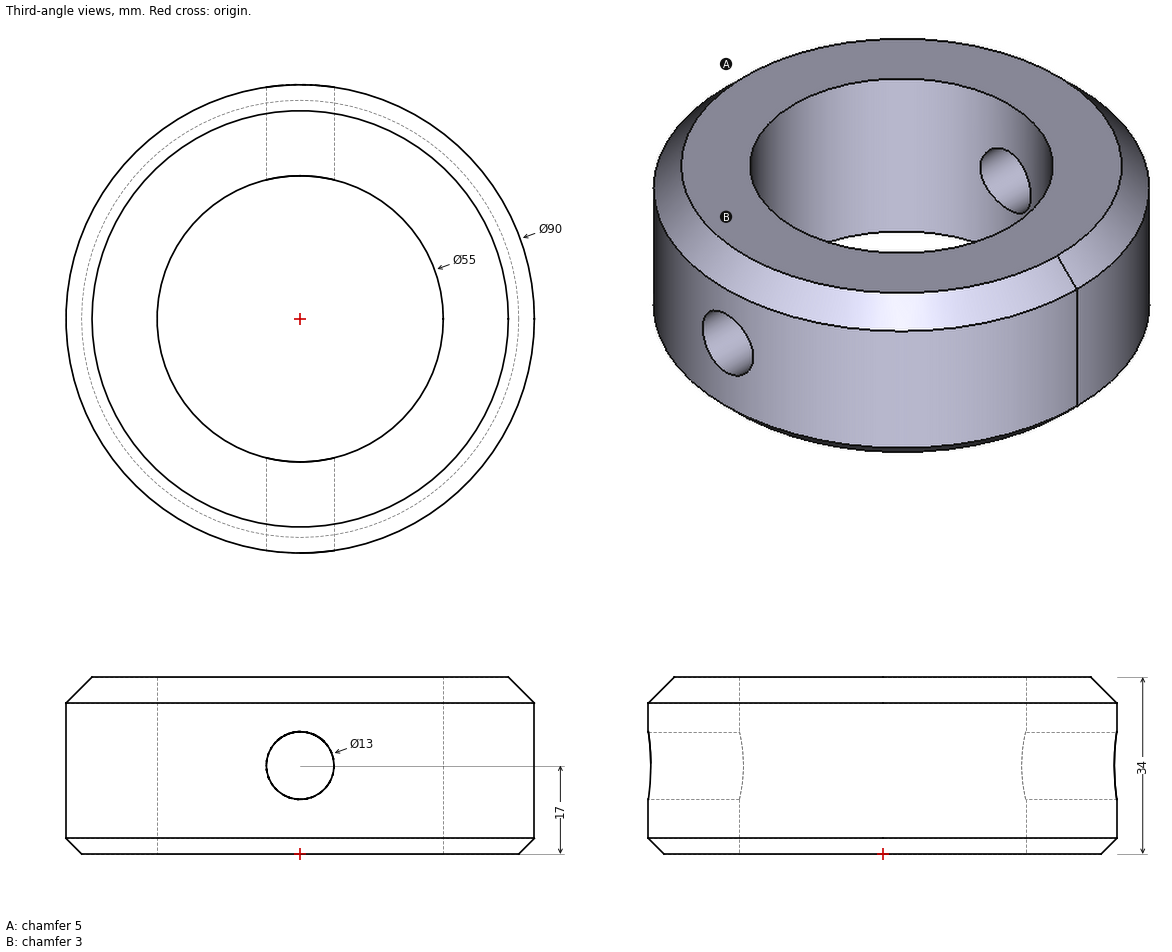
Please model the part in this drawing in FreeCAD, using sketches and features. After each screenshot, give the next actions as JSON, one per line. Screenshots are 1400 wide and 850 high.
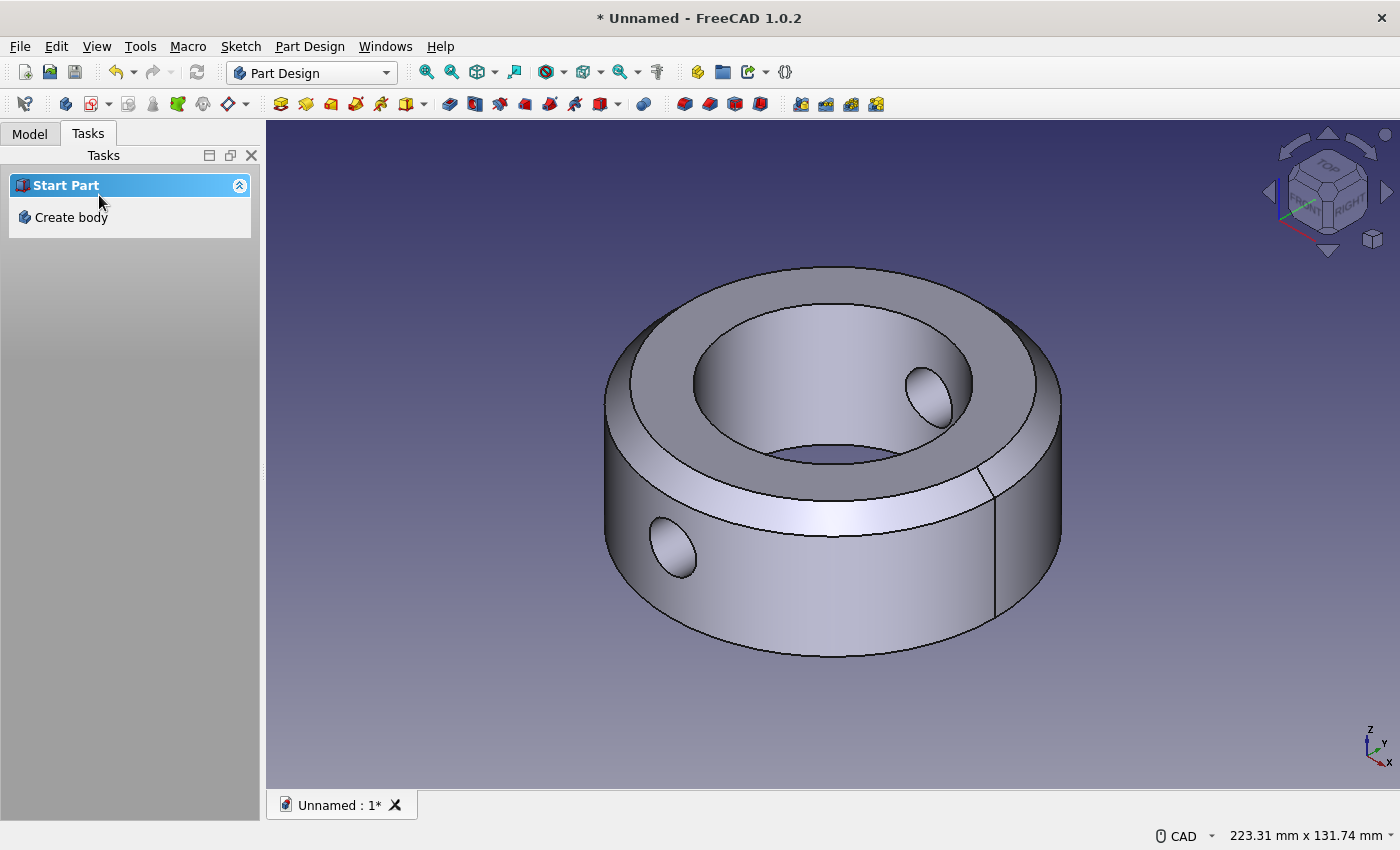
{"action": "left_click", "coordinate": [729, 642]}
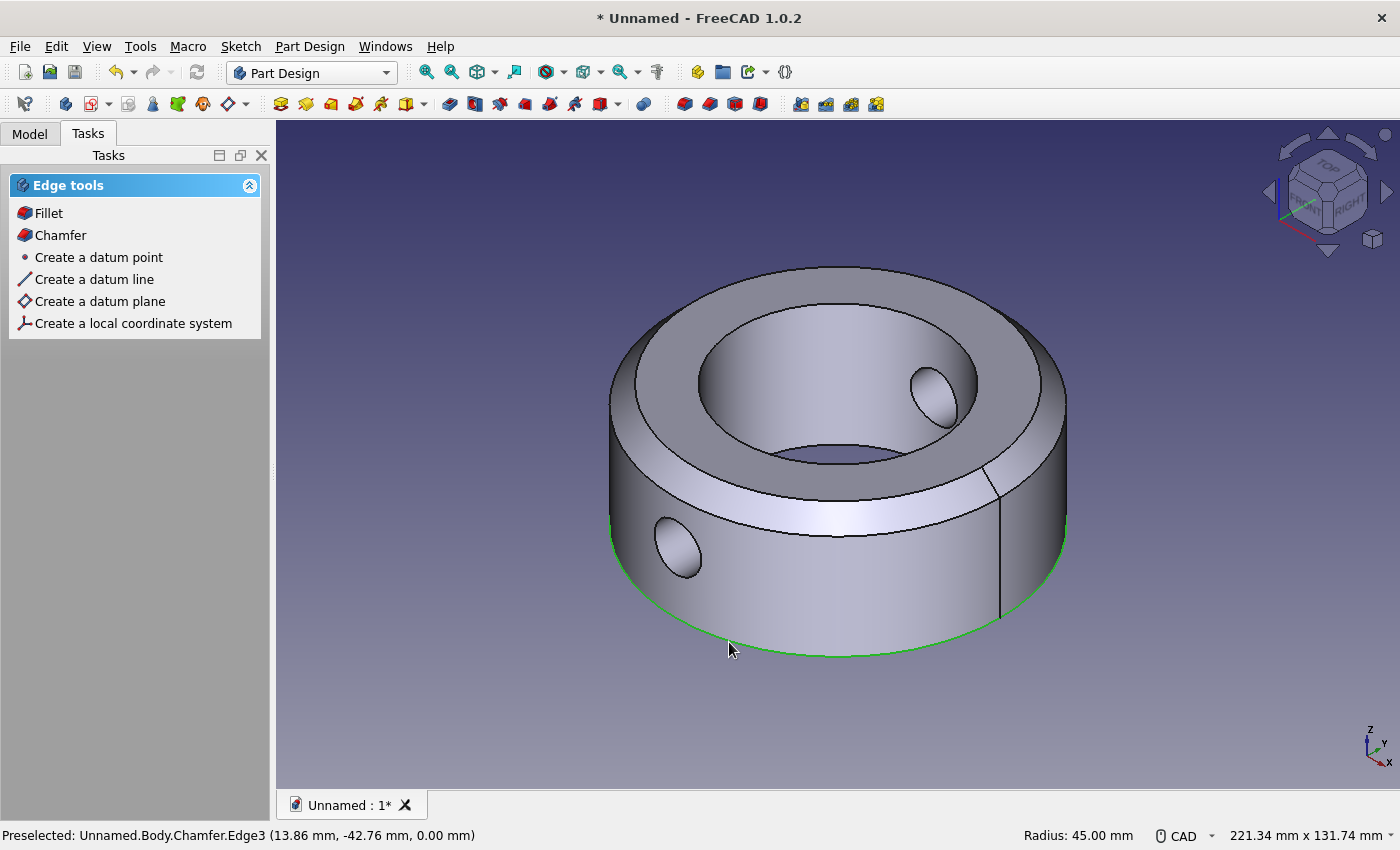
{"action": "left_click", "coordinate": [710, 104]}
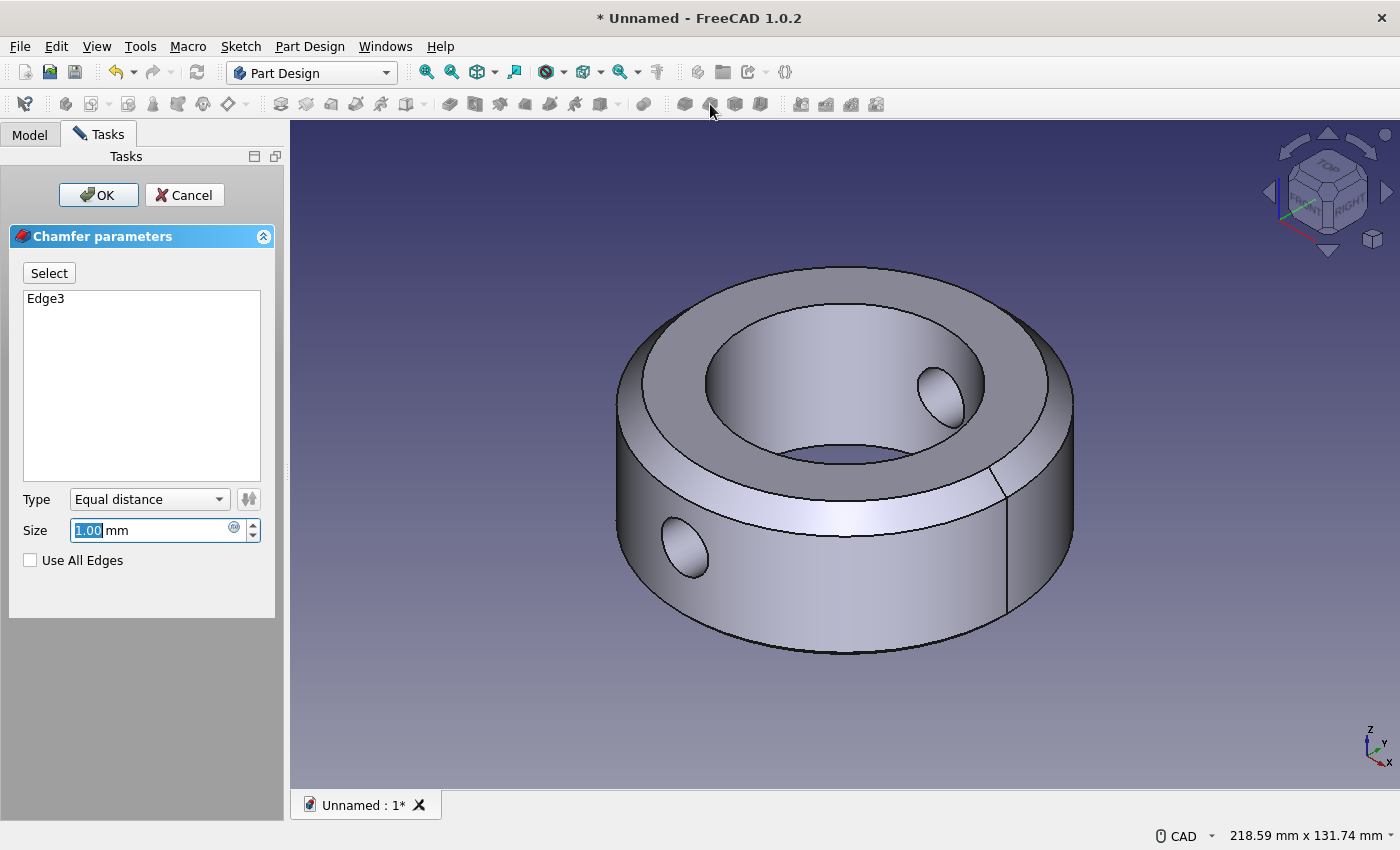
{"action": "type", "text": "3"}
{"action": "key", "text": "Tab"}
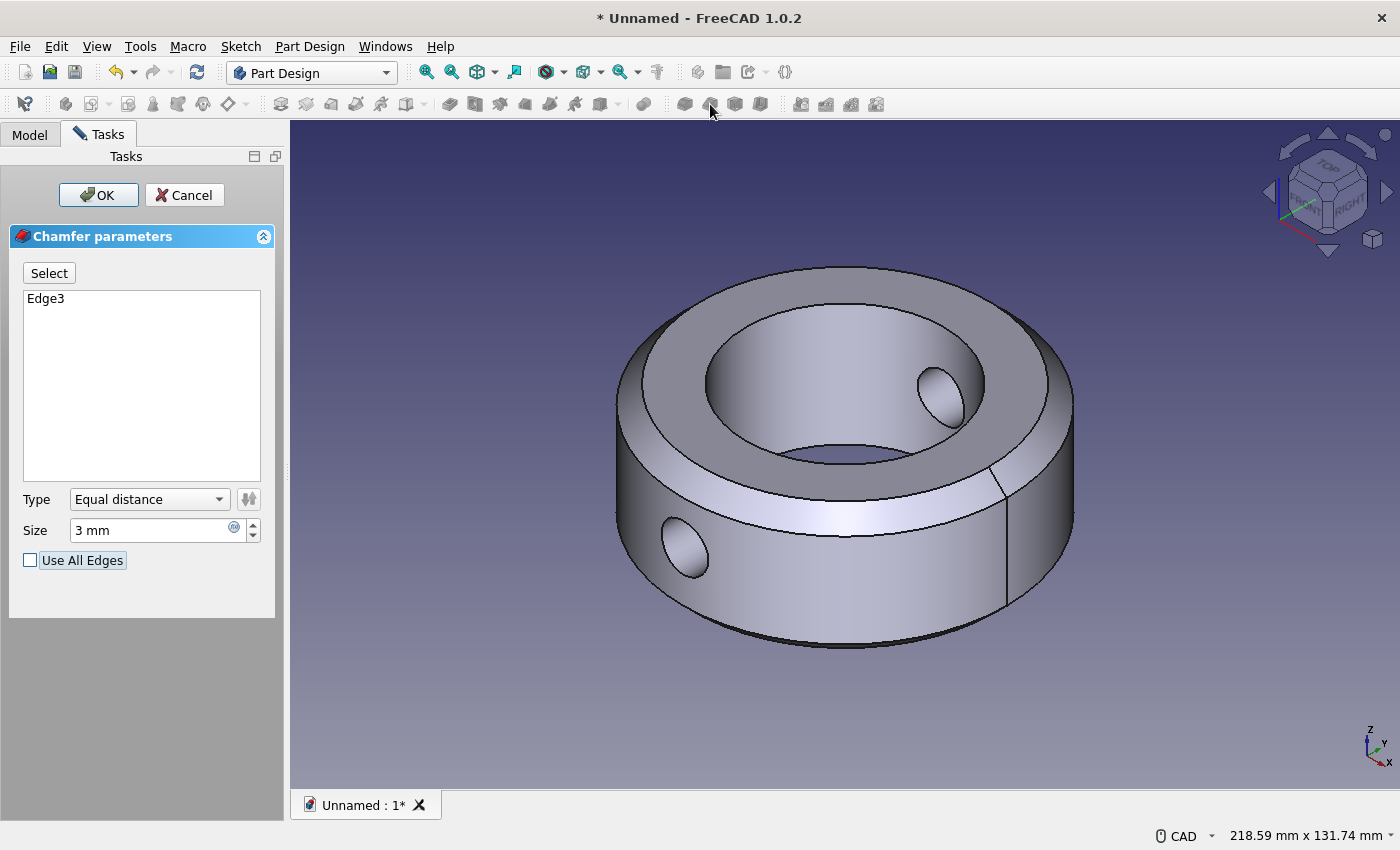
{"action": "left_click", "coordinate": [99, 195]}